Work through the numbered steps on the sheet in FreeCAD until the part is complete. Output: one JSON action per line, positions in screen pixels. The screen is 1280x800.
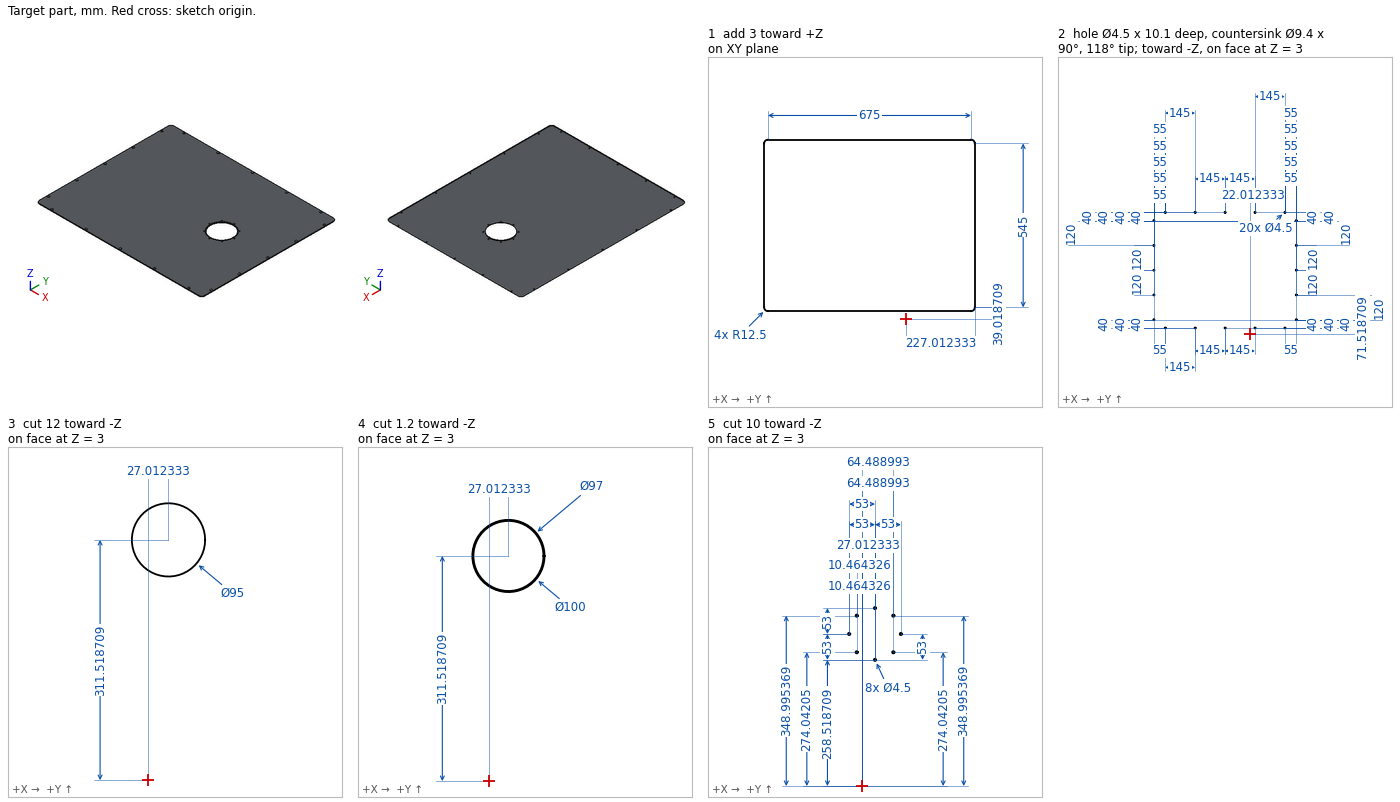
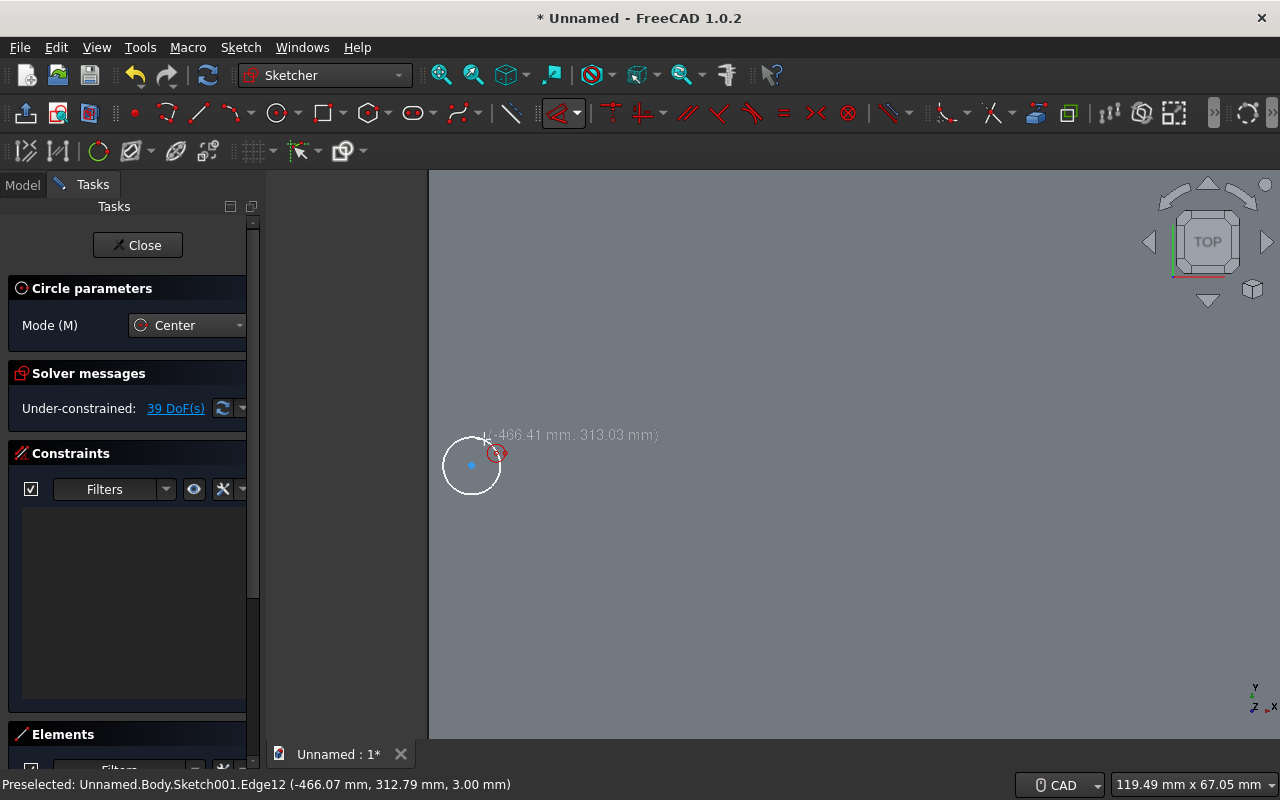
{"action": "scroll", "coordinate": [488, 445], "scroll_direction": "down", "scroll_amount": 13}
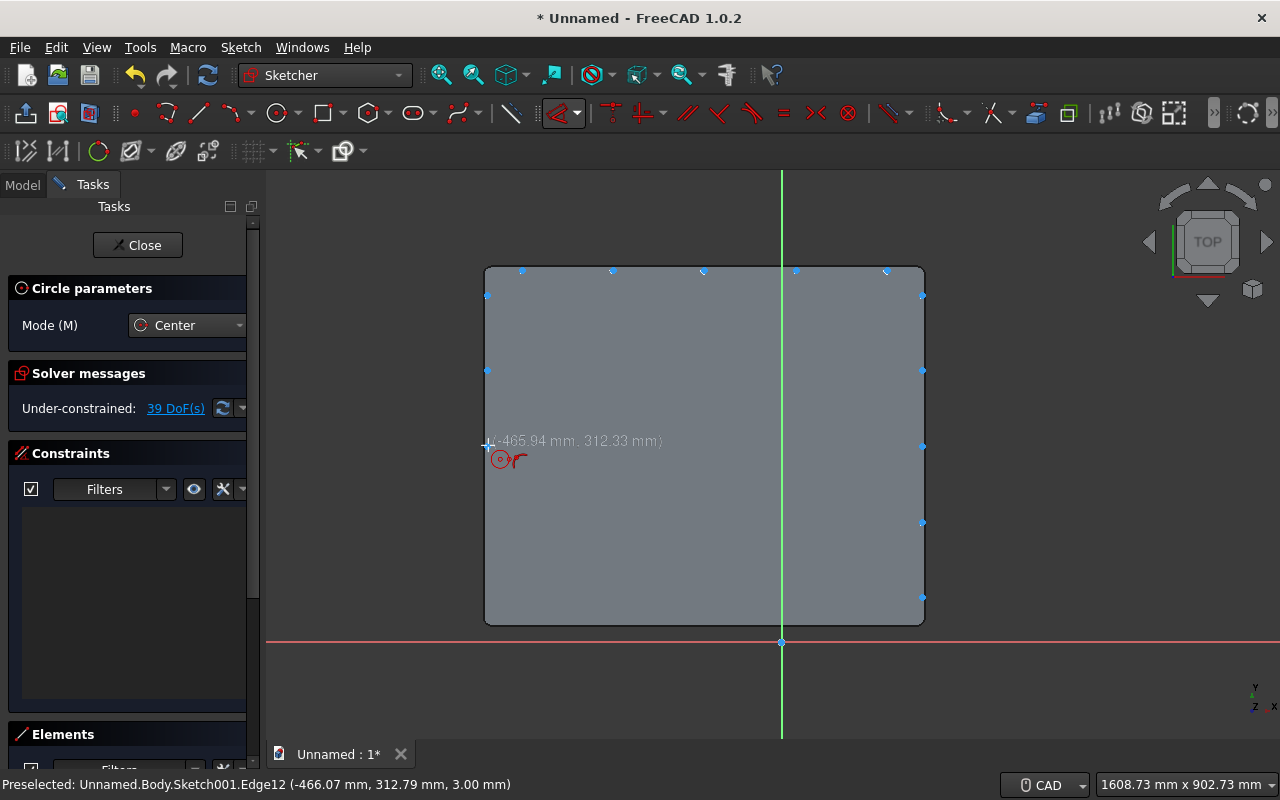
{"action": "scroll", "coordinate": [487, 522], "scroll_direction": "up", "scroll_amount": 14}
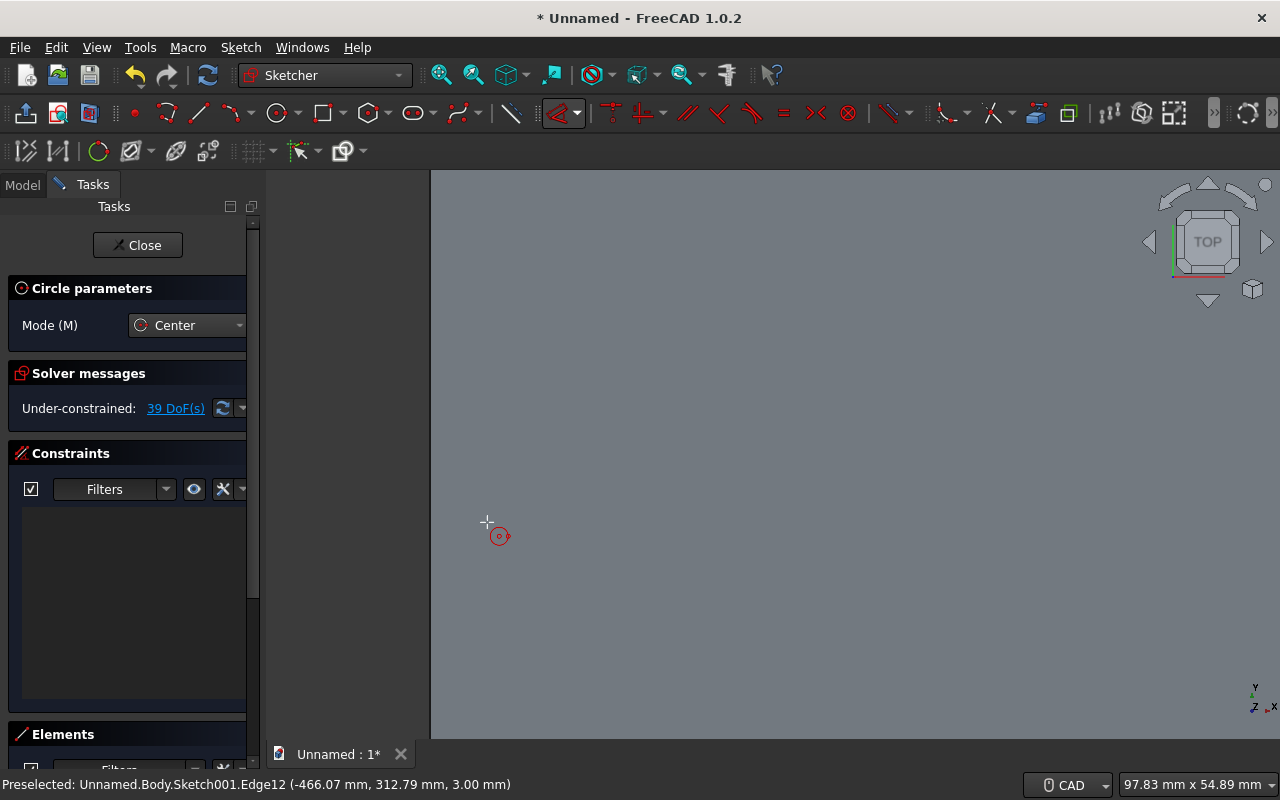
{"action": "scroll", "coordinate": [487, 522], "scroll_direction": "down", "scroll_amount": 14}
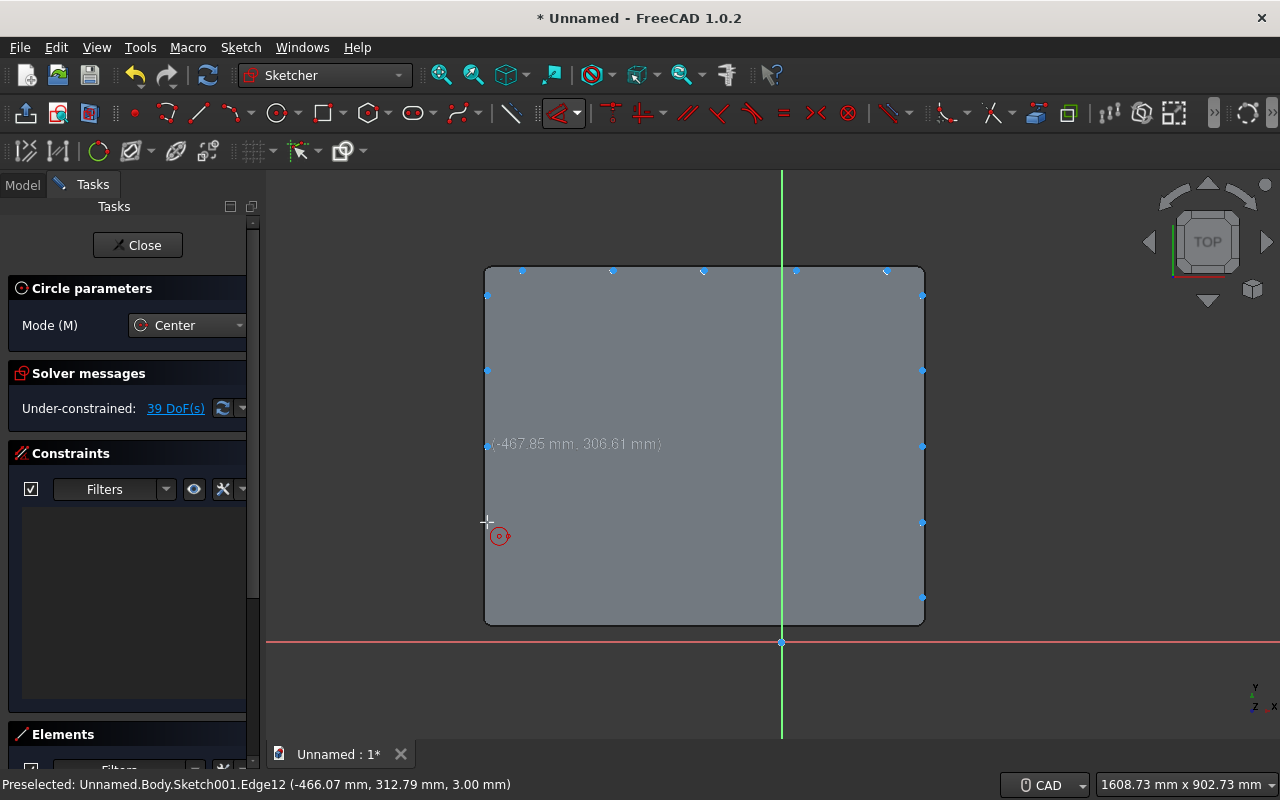
{"action": "left_click", "coordinate": [487, 522]}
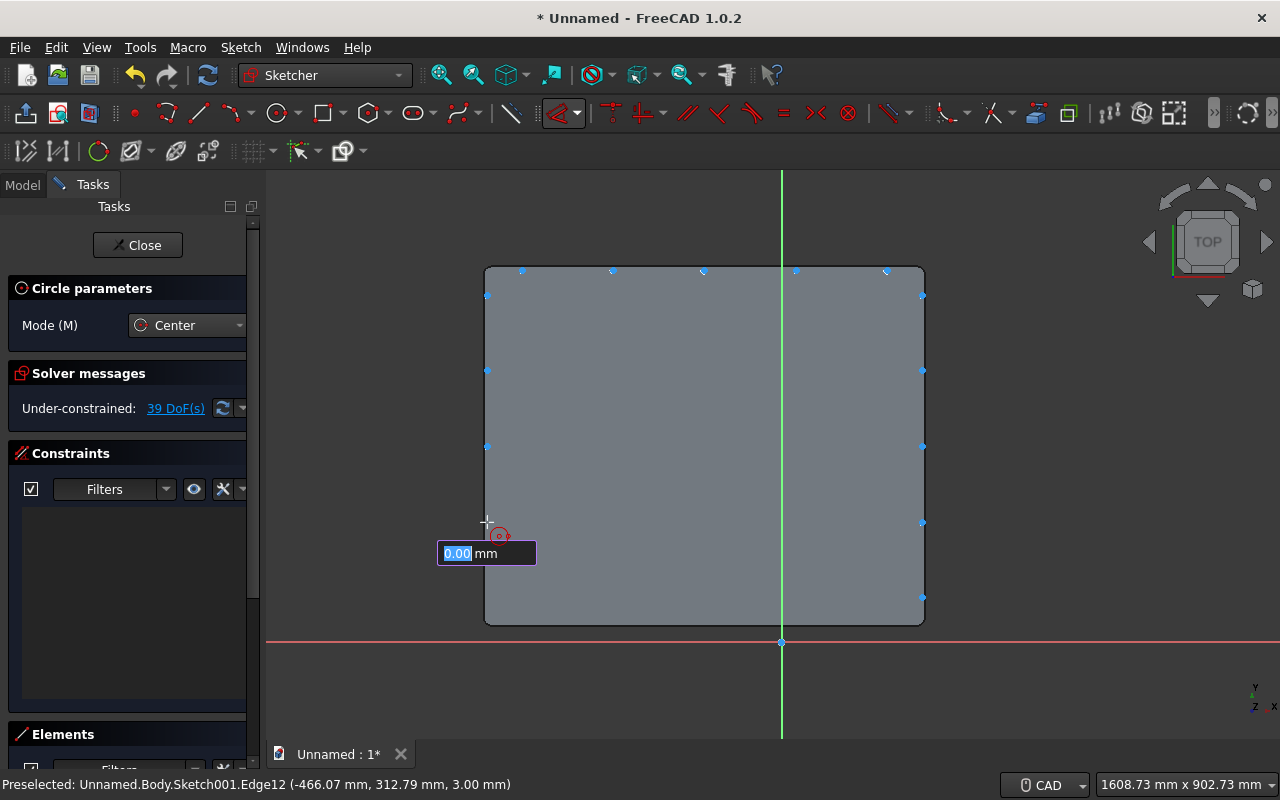
{"action": "scroll", "coordinate": [488, 521], "scroll_direction": "up", "scroll_amount": 13}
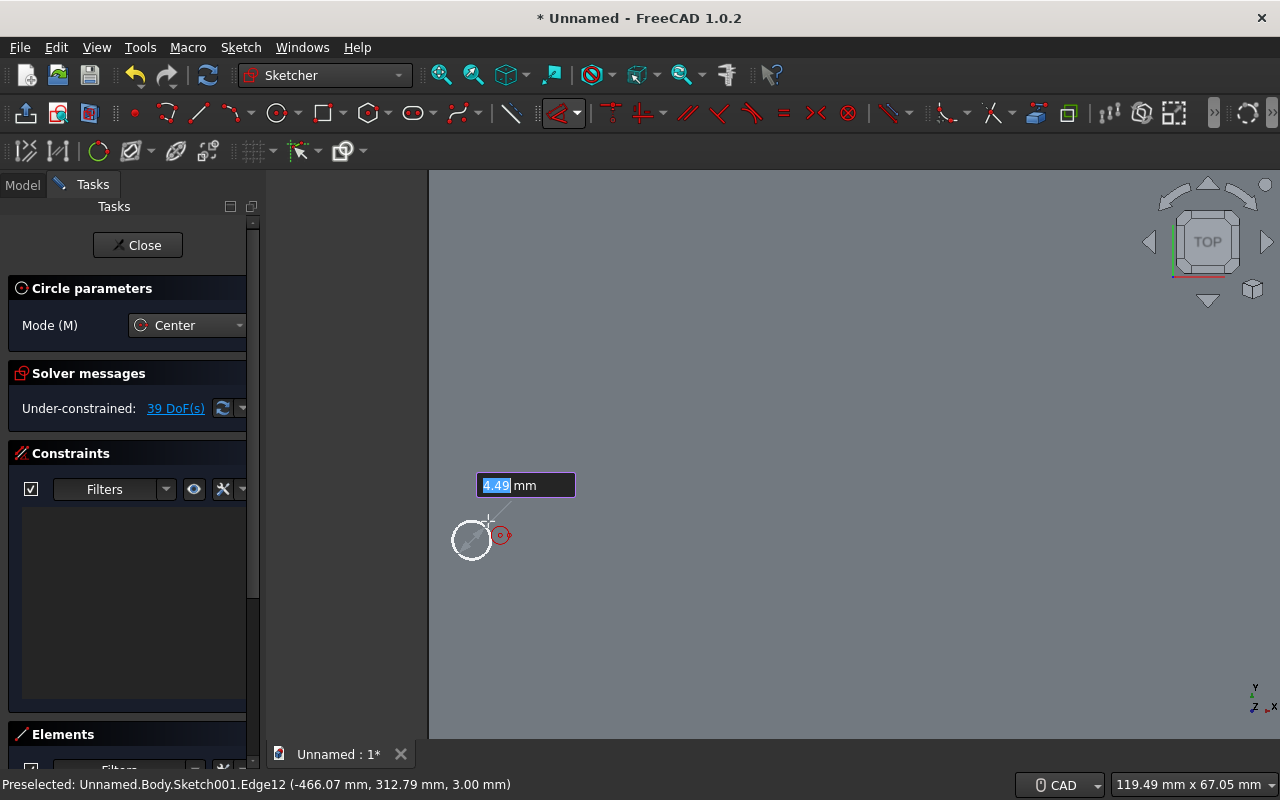
{"action": "left_click", "coordinate": [484, 509]}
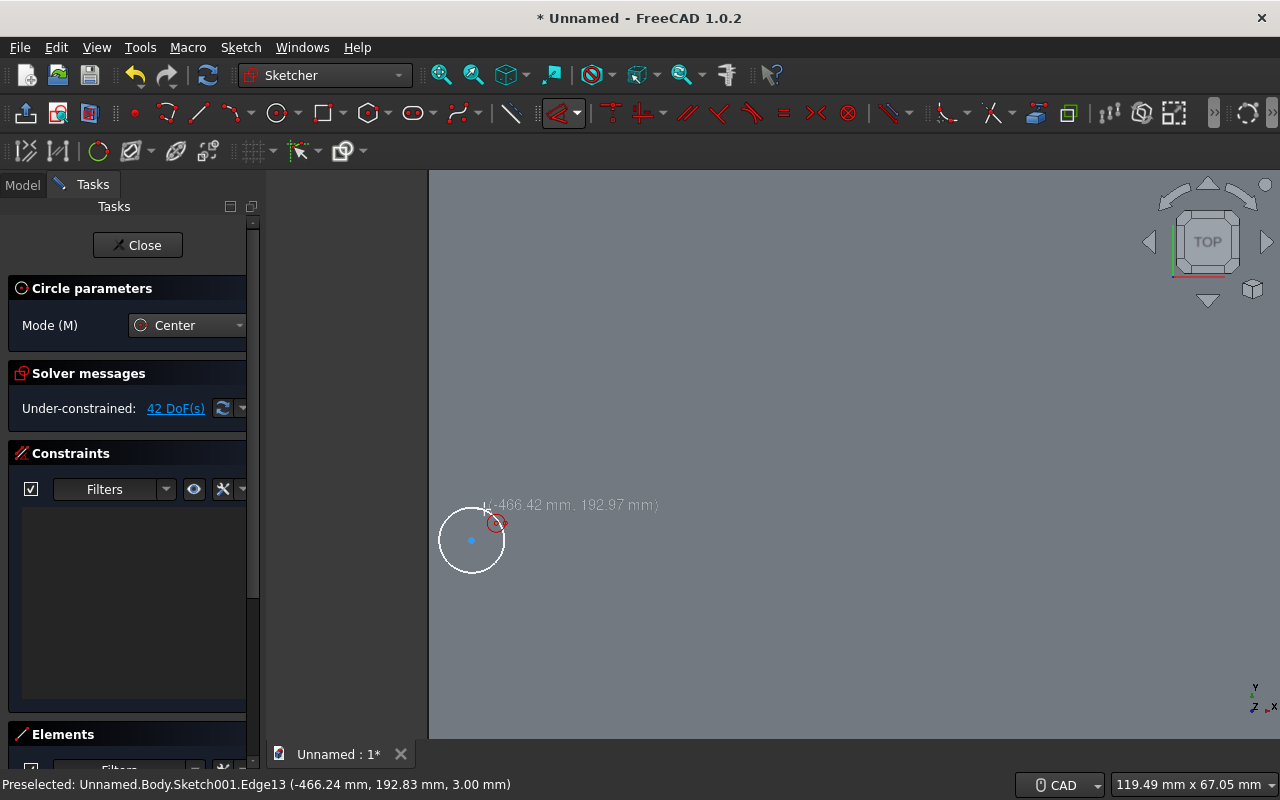
{"action": "scroll", "coordinate": [488, 521], "scroll_direction": "down", "scroll_amount": 13}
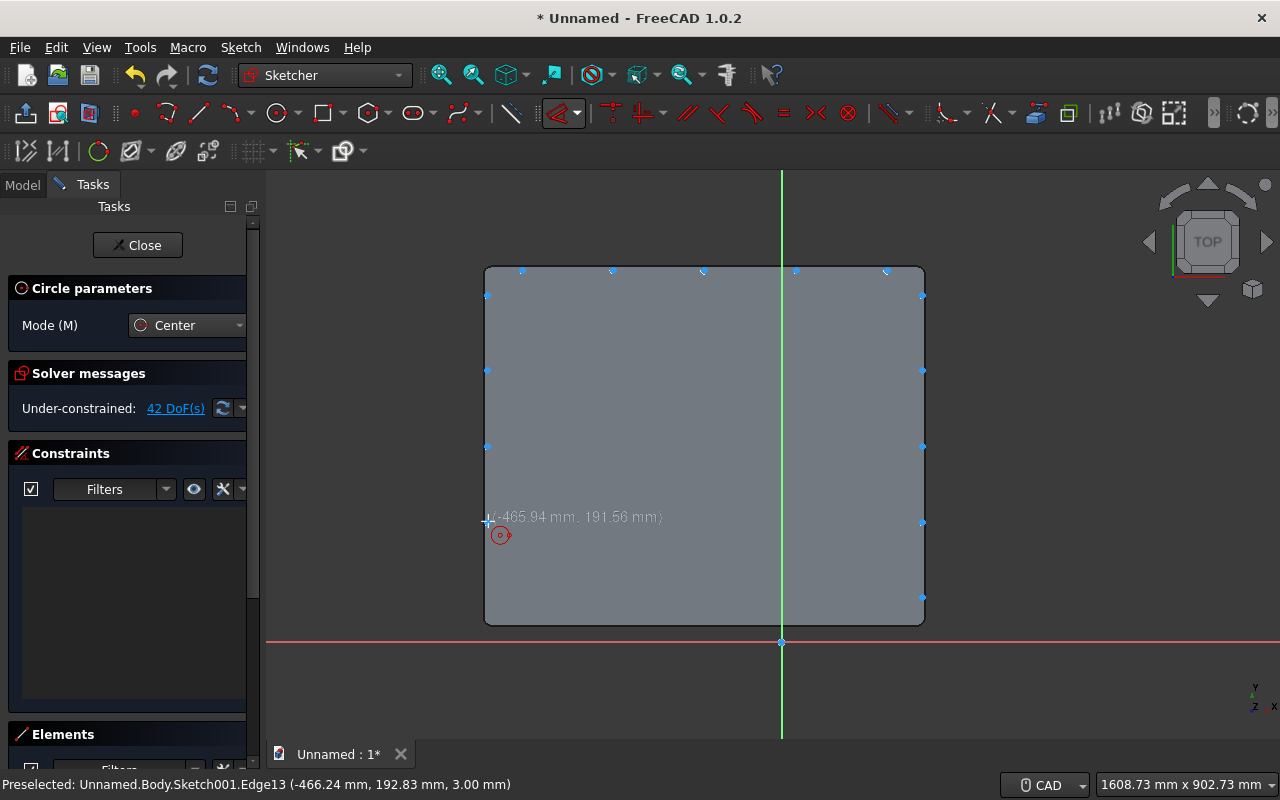
{"action": "scroll", "coordinate": [487, 597], "scroll_direction": "up", "scroll_amount": 14}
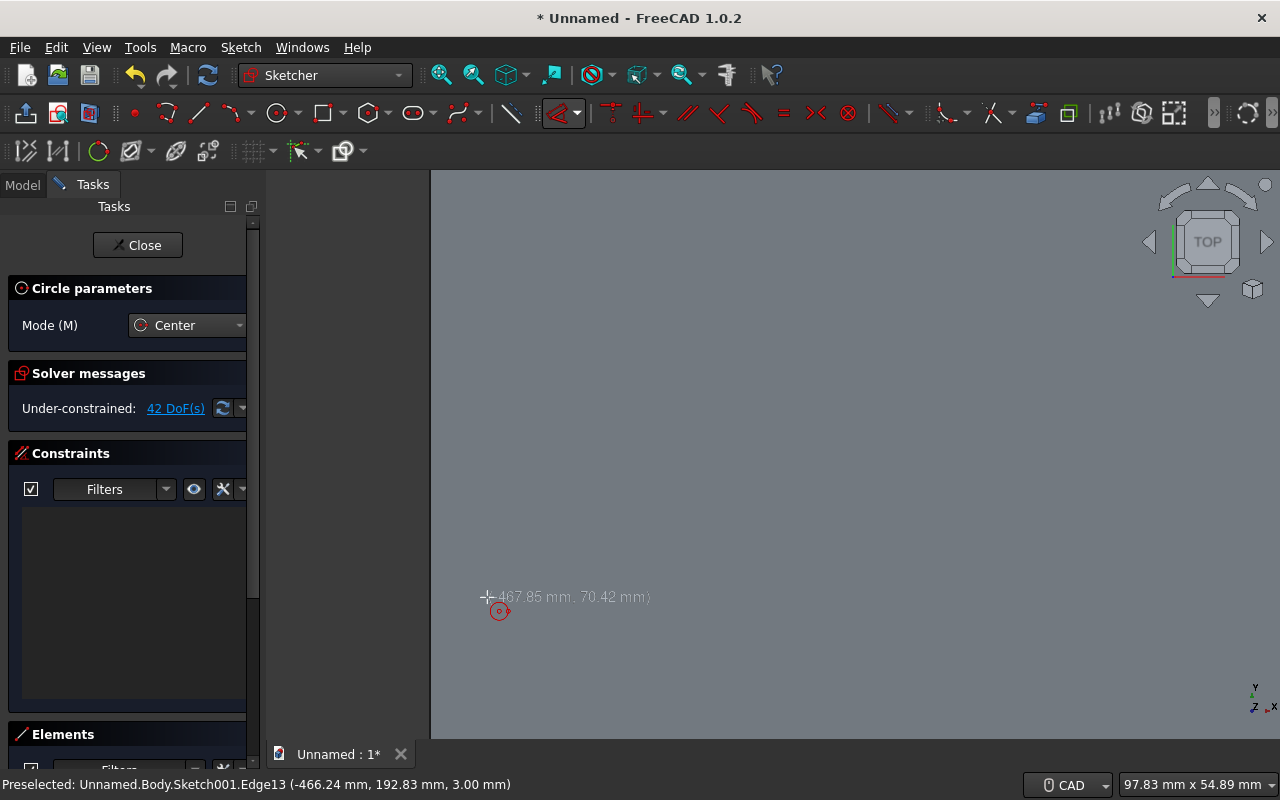
{"action": "scroll", "coordinate": [487, 597], "scroll_direction": "down", "scroll_amount": 14}